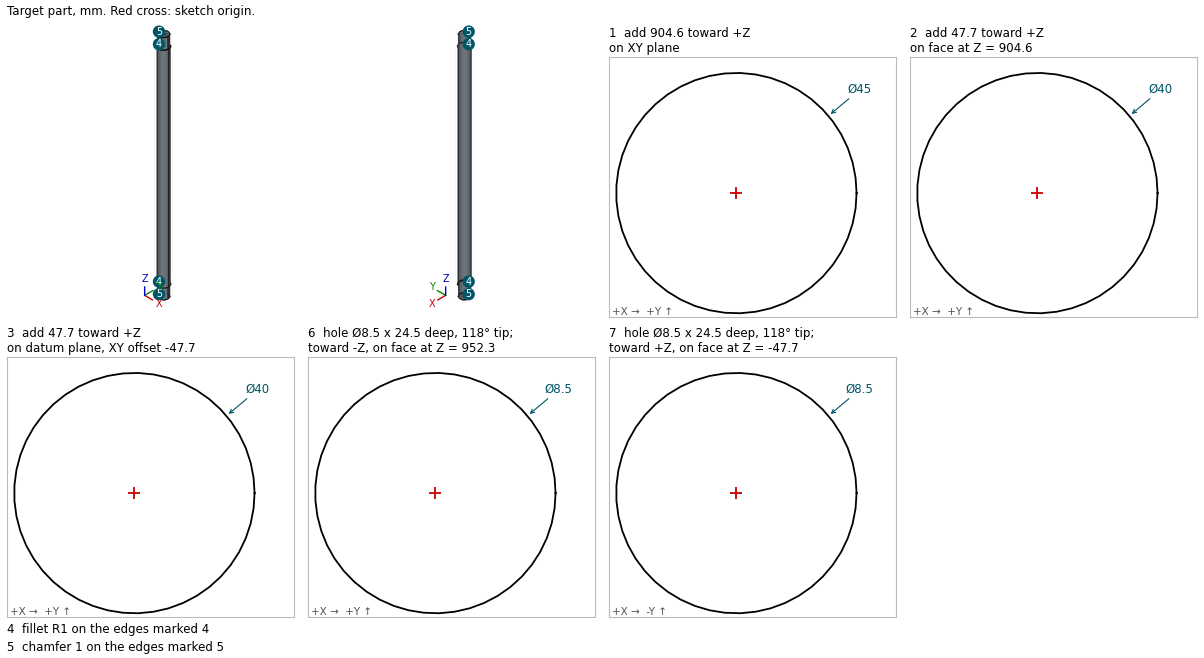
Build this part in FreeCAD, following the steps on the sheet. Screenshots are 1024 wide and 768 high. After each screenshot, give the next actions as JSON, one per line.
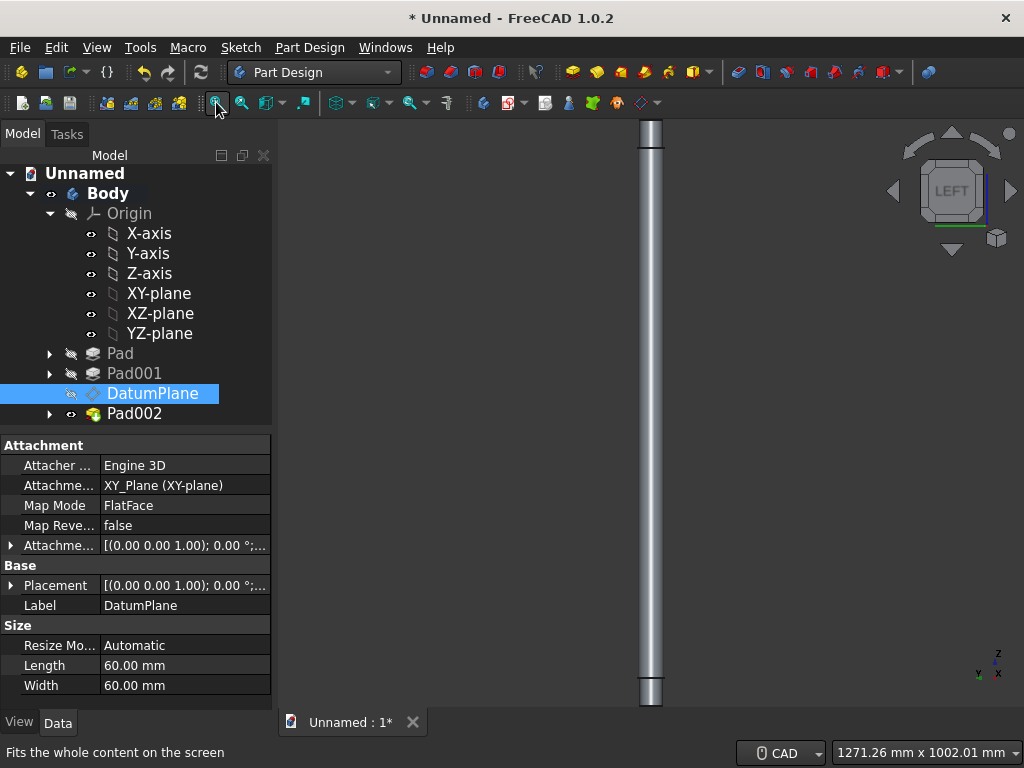
{"action": "key", "text": "0"}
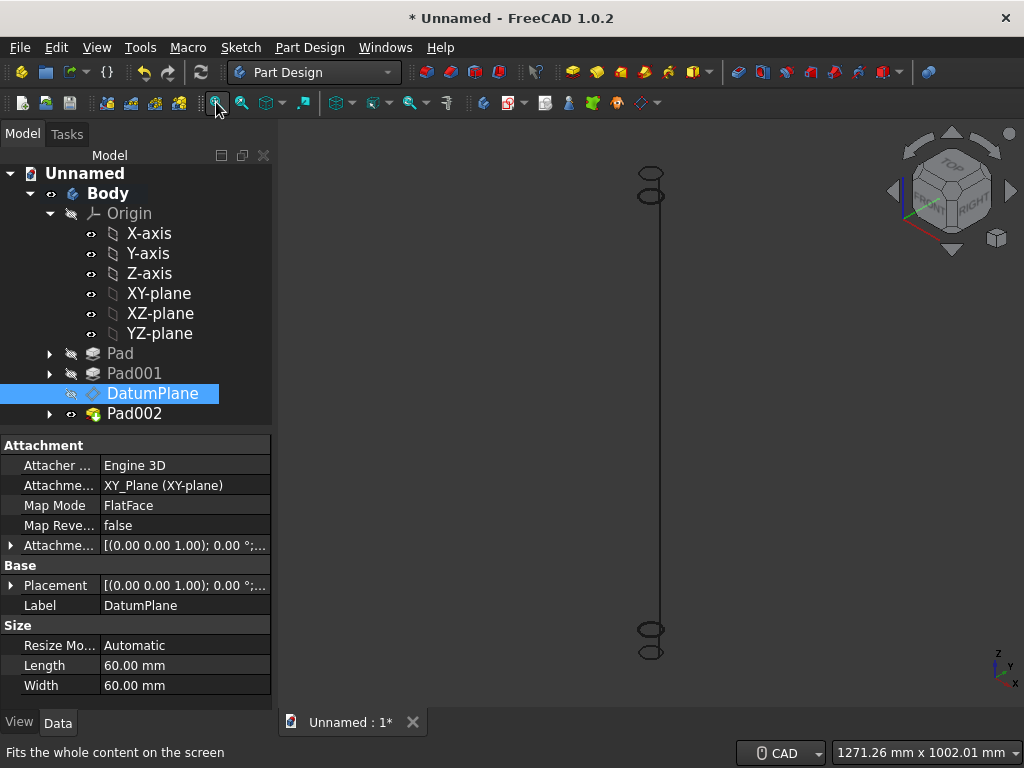
{"action": "left_click", "coordinate": [643, 190]}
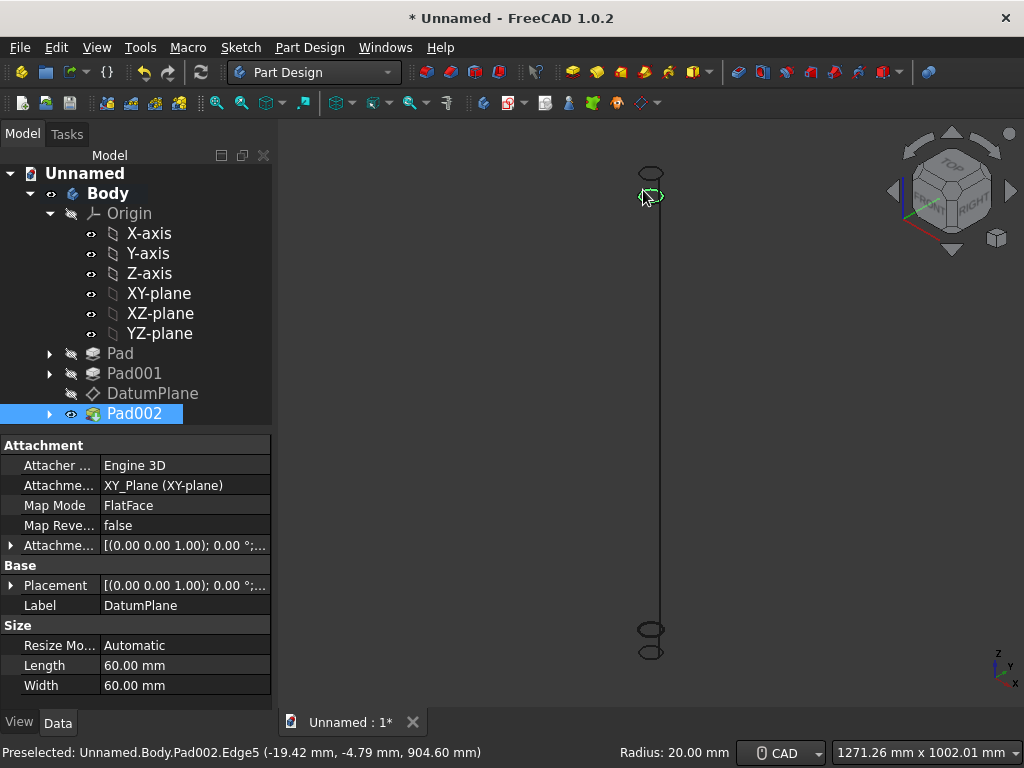
{"action": "left_click", "coordinate": [643, 624], "text": "ctrl"}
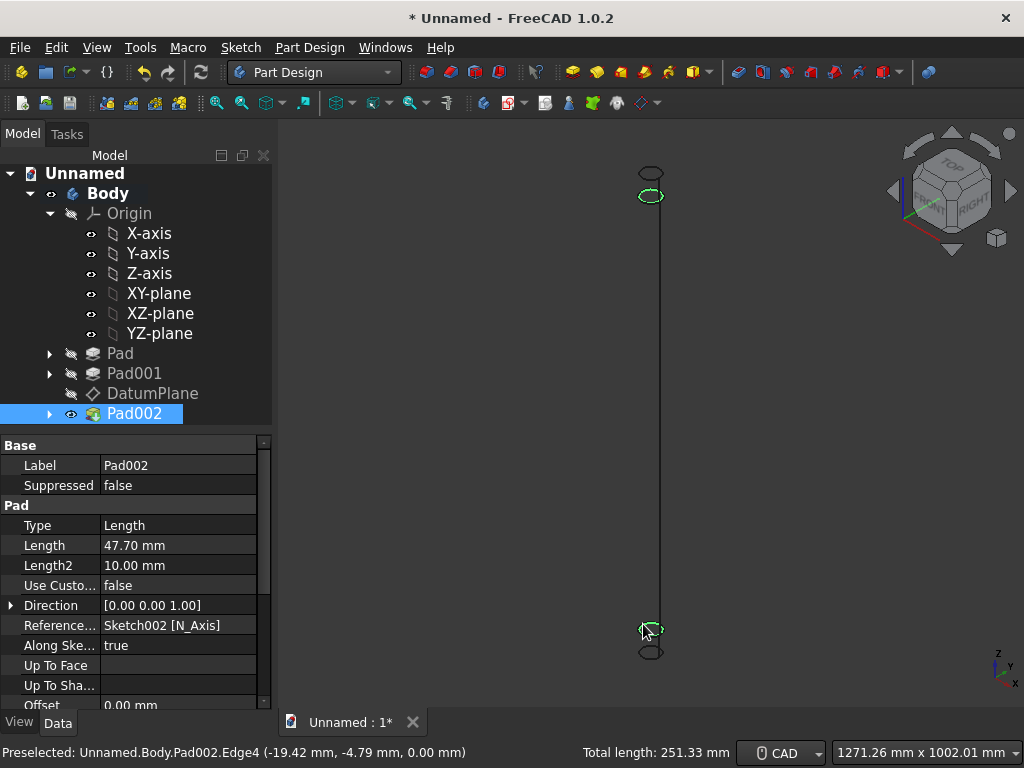
{"action": "key", "text": "v 1"}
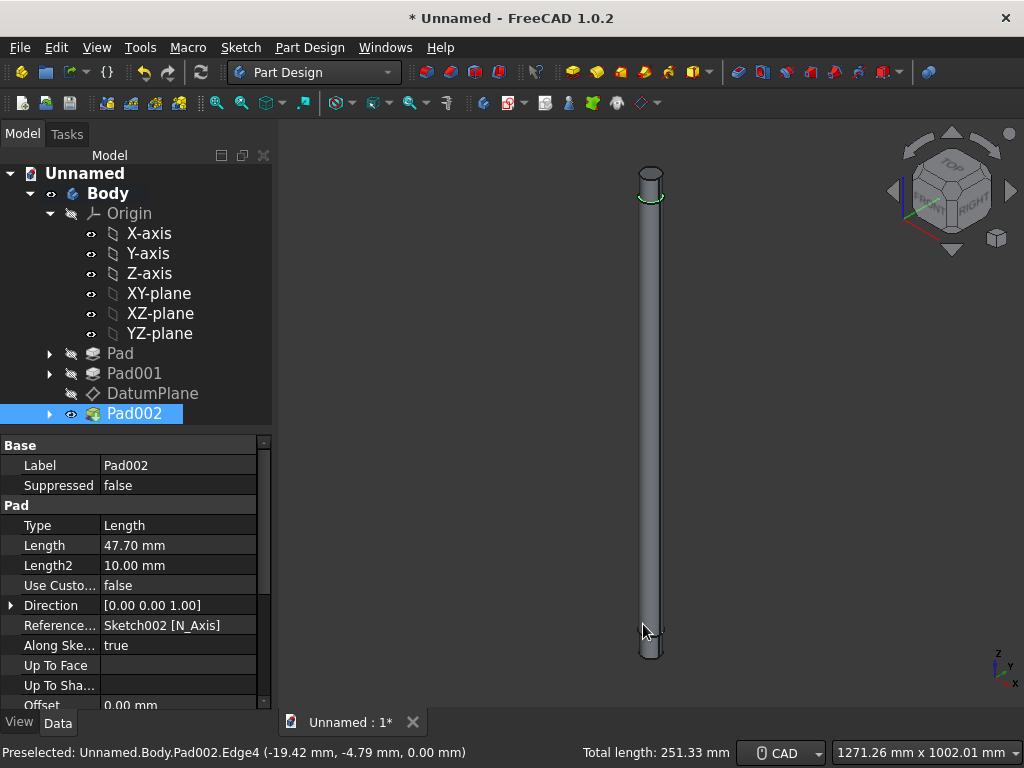
{"action": "left_click", "coordinate": [428, 72]}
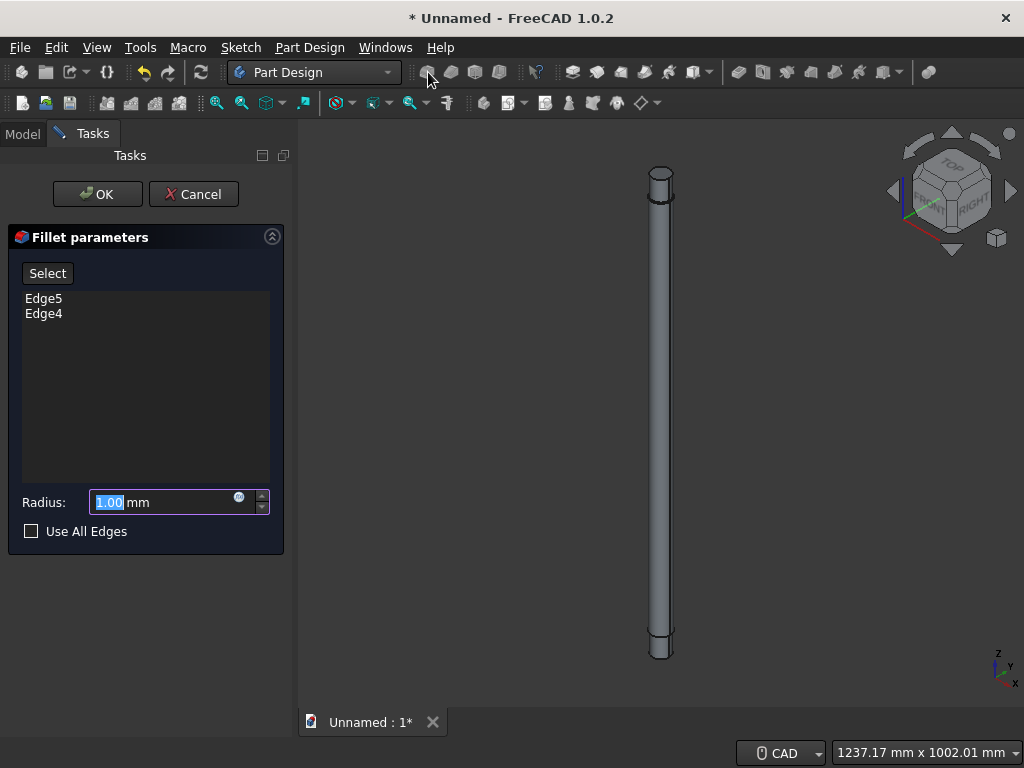
{"action": "type", "text": "1"}
{"action": "key", "text": "Tab"}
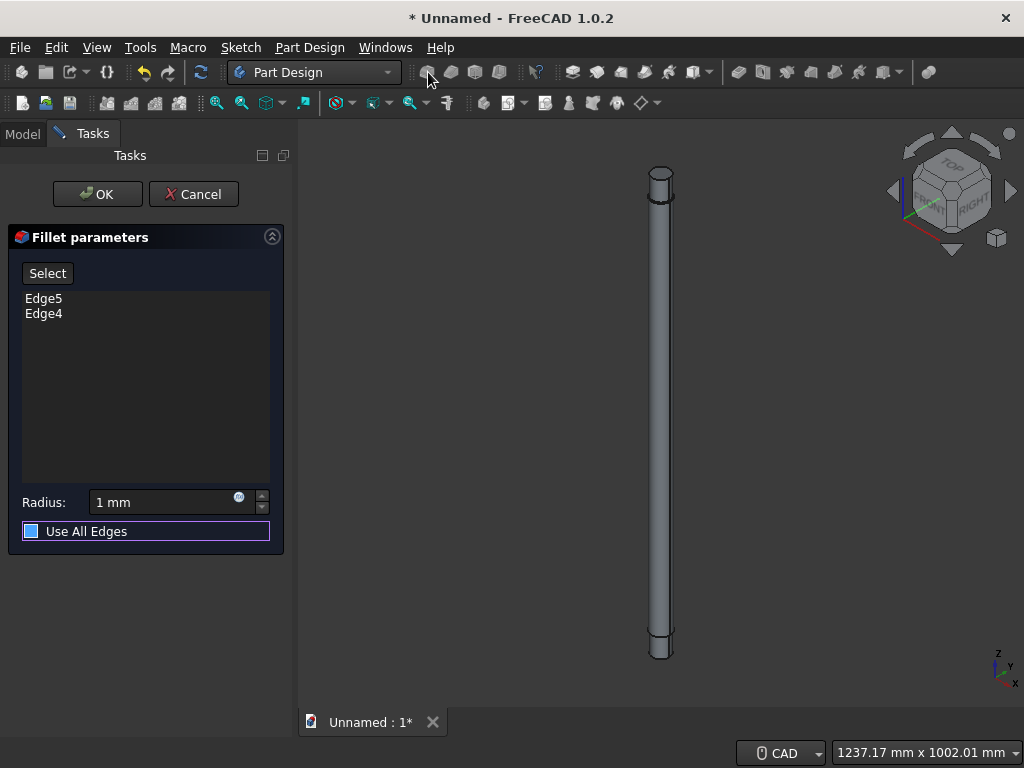
{"action": "left_click", "coordinate": [98, 194]}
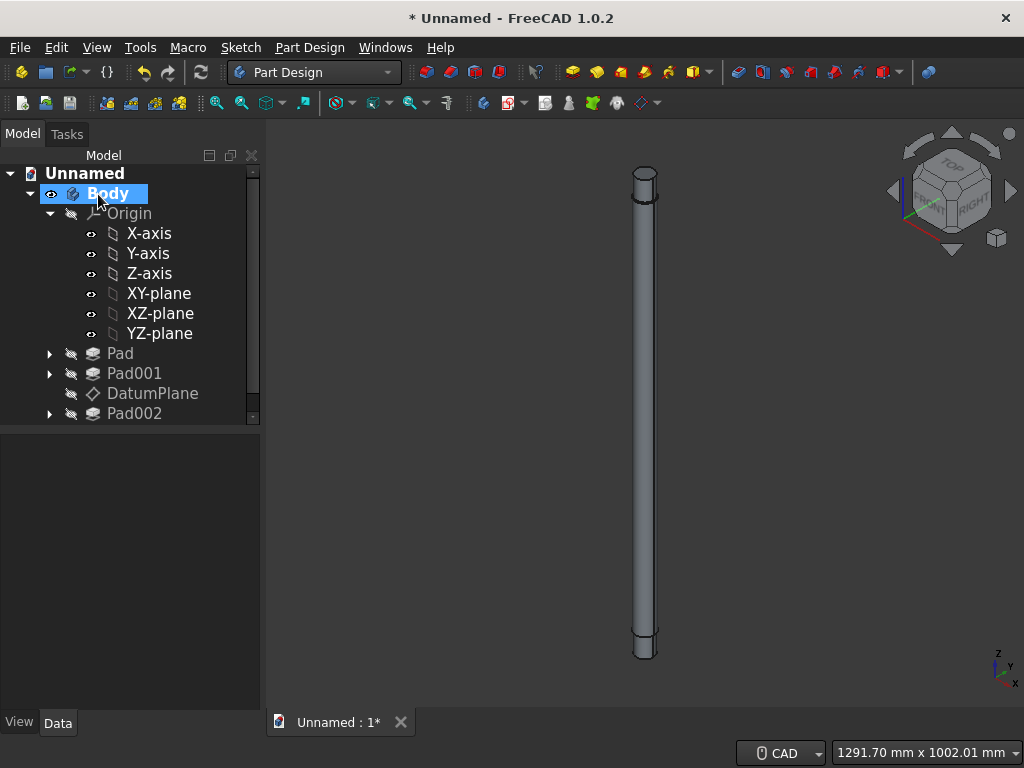
{"action": "left_click", "coordinate": [635, 655]}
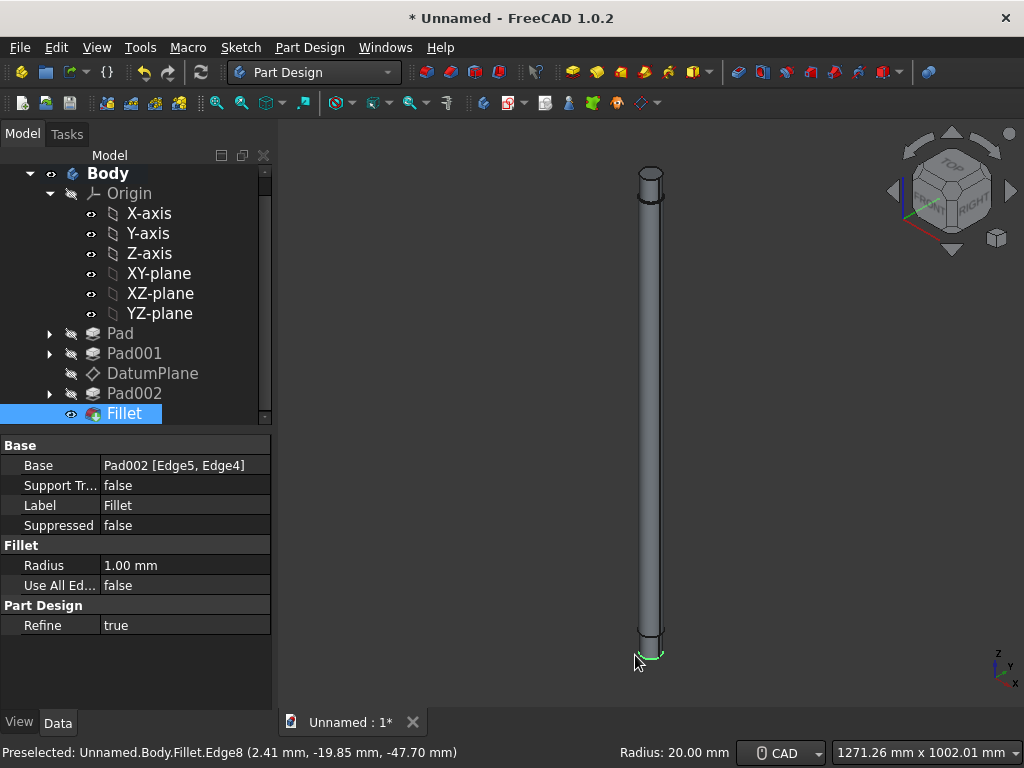
{"action": "left_click", "coordinate": [639, 171], "text": "ctrl"}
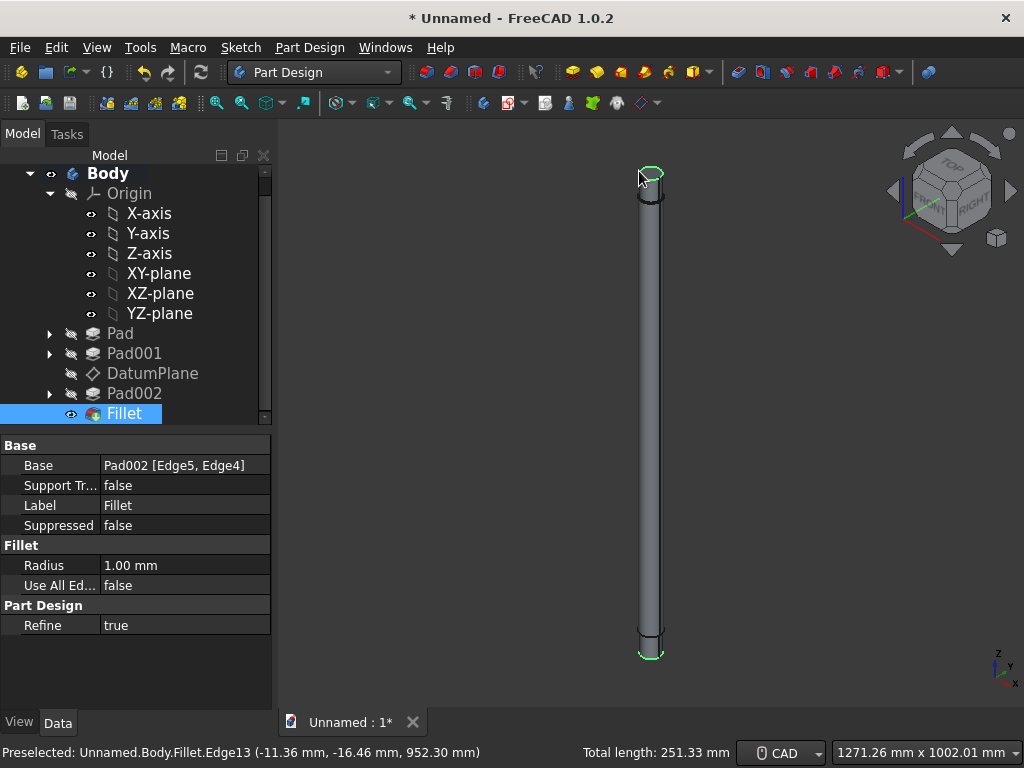
{"action": "left_click", "coordinate": [452, 72]}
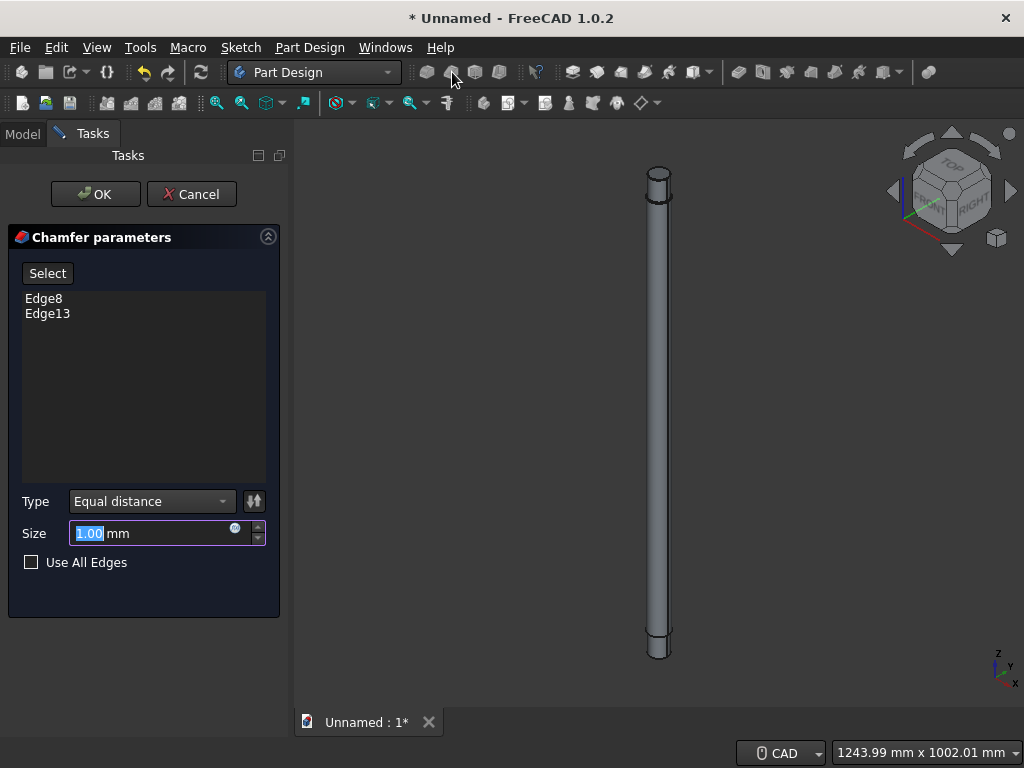
{"action": "type", "text": "1"}
{"action": "key", "text": "Tab"}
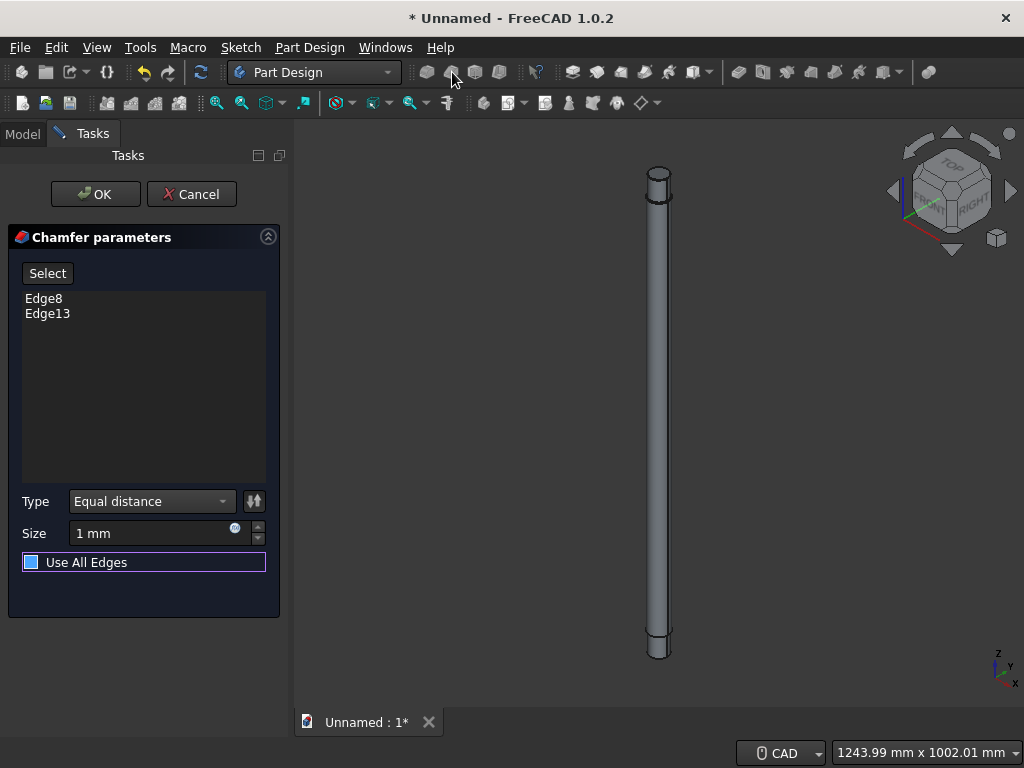
{"action": "left_click", "coordinate": [96, 194]}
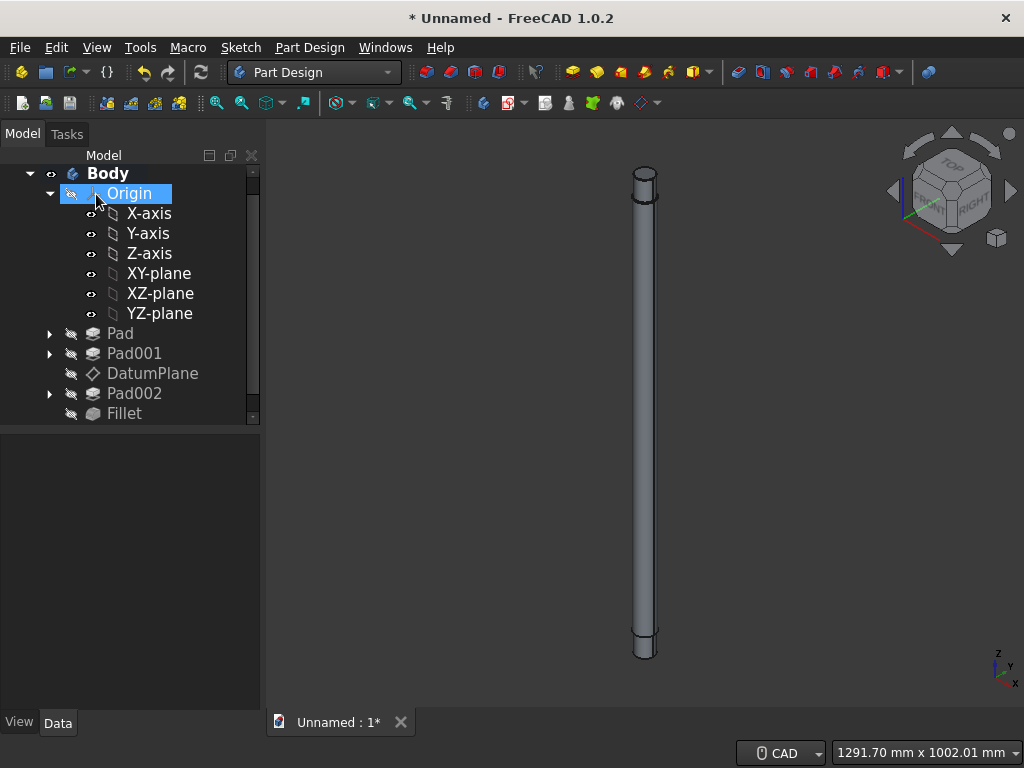
{"action": "key", "text": "2"}